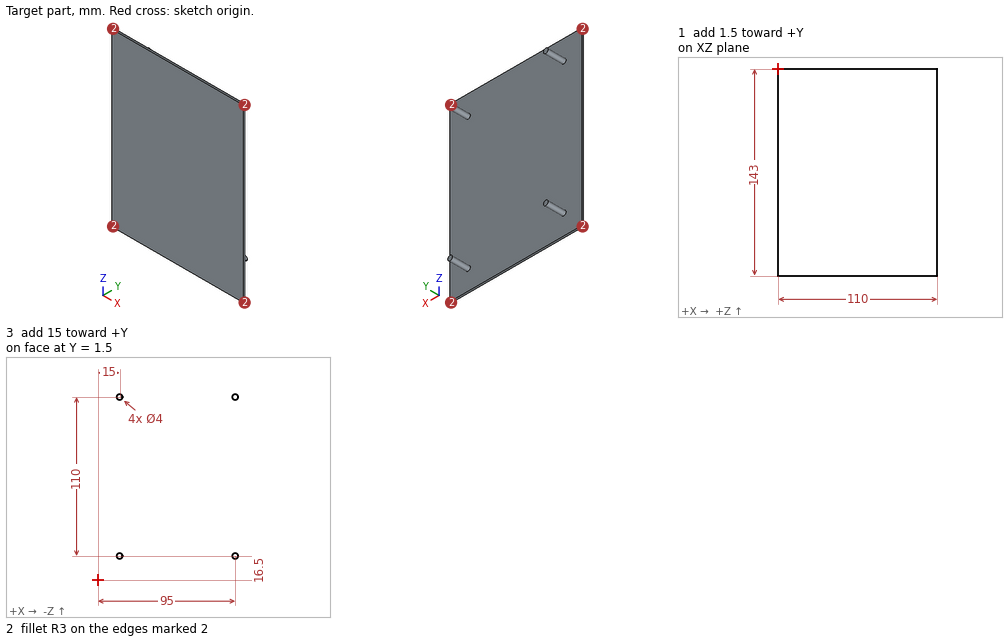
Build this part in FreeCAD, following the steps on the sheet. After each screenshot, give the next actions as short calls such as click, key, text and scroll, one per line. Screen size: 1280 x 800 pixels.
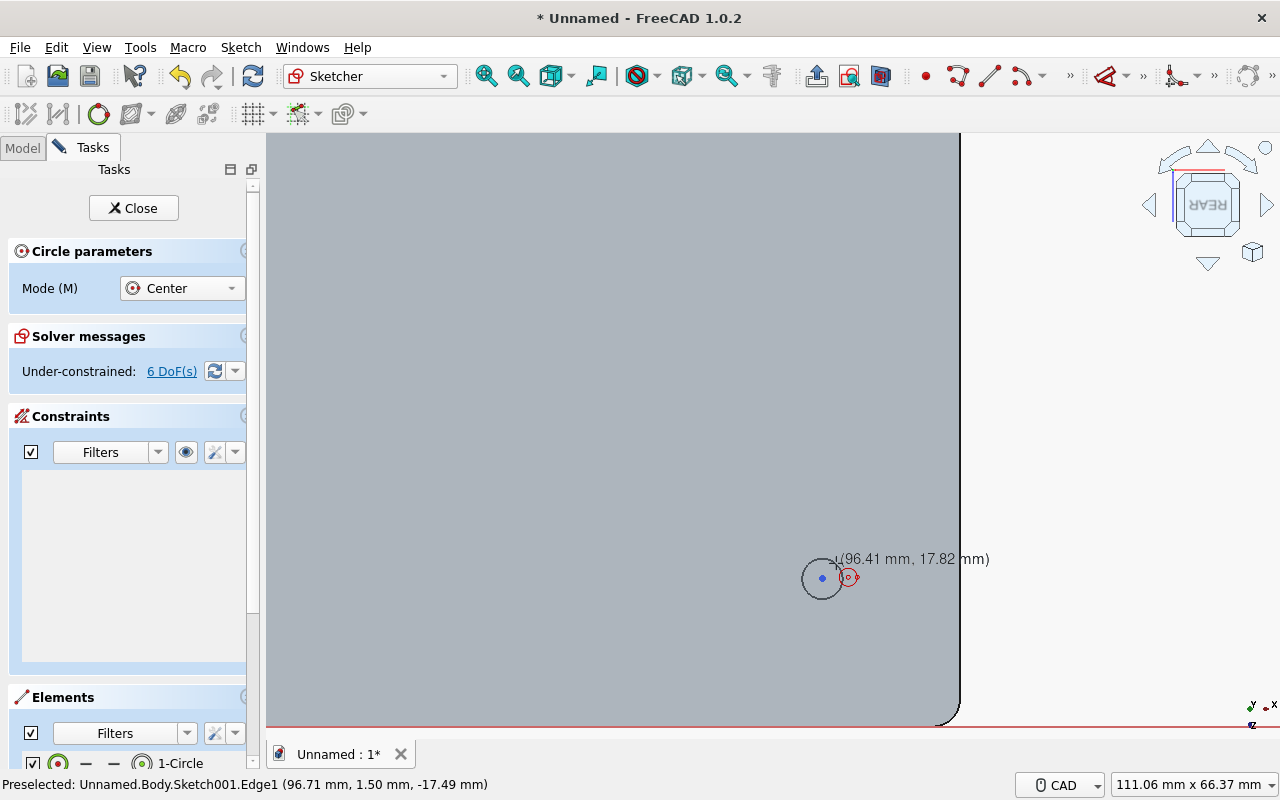
scroll(836, 564, down, 6)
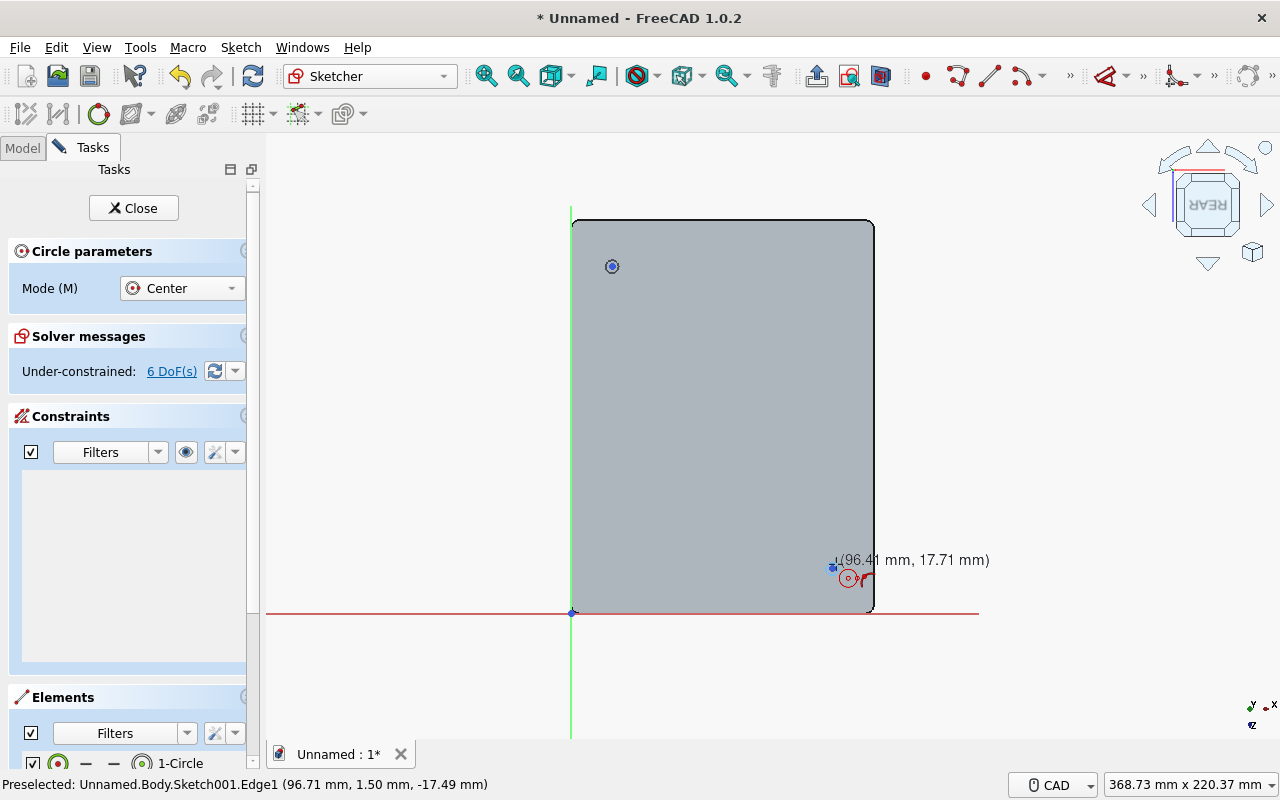
scroll(613, 568, up, 8)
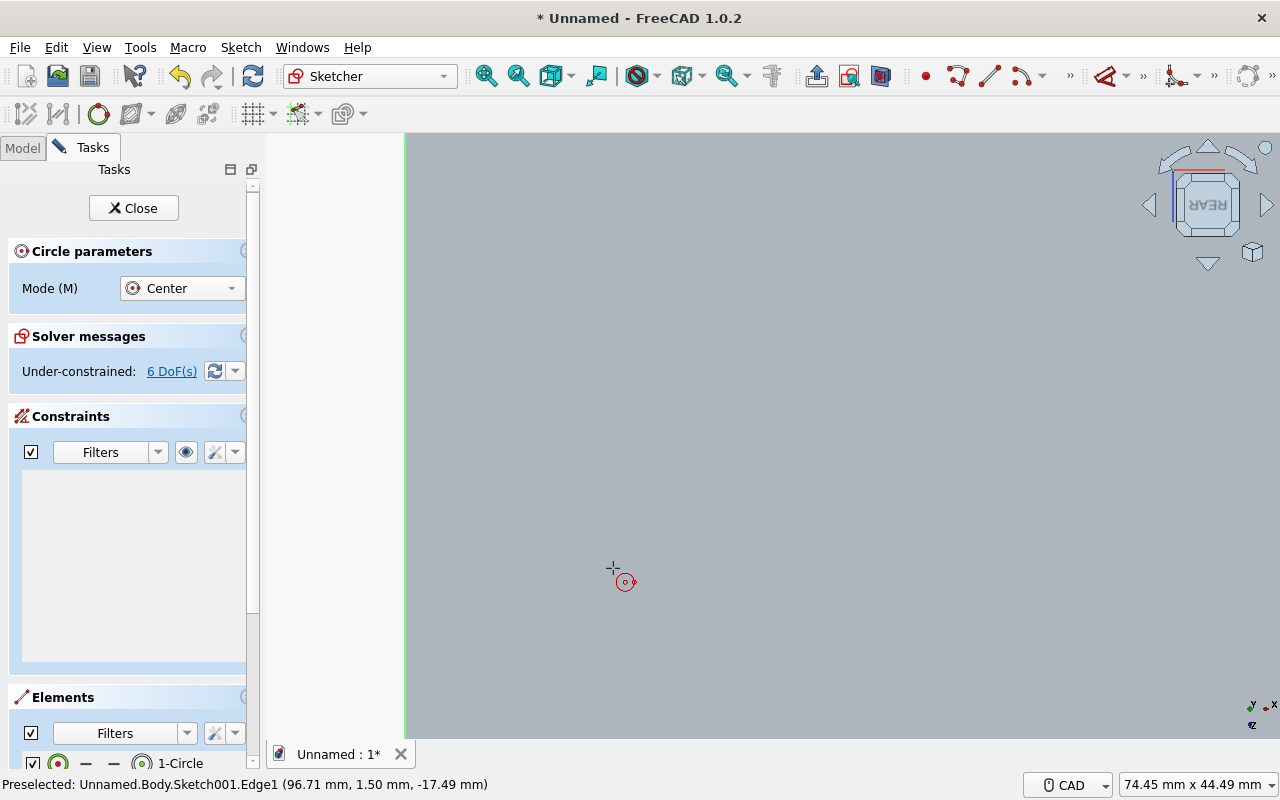
scroll(613, 568, down, 8)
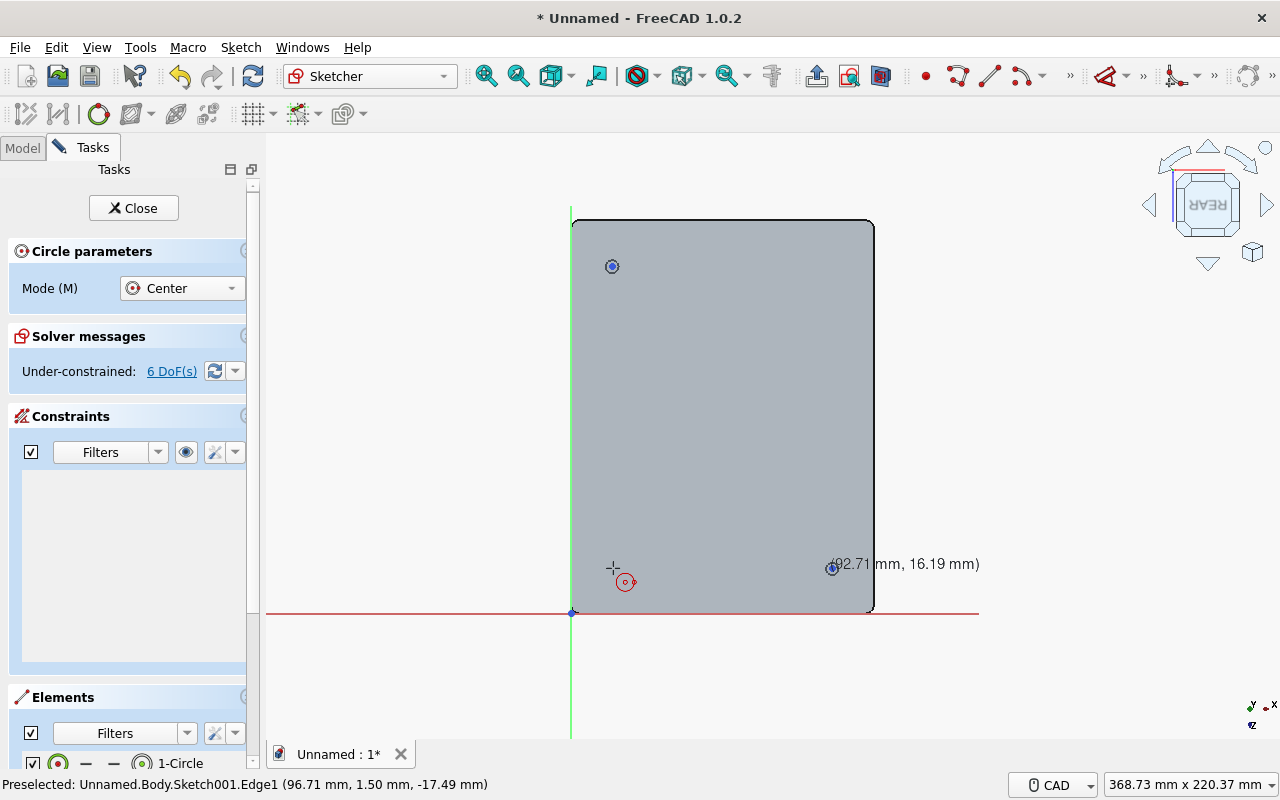
click(613, 568)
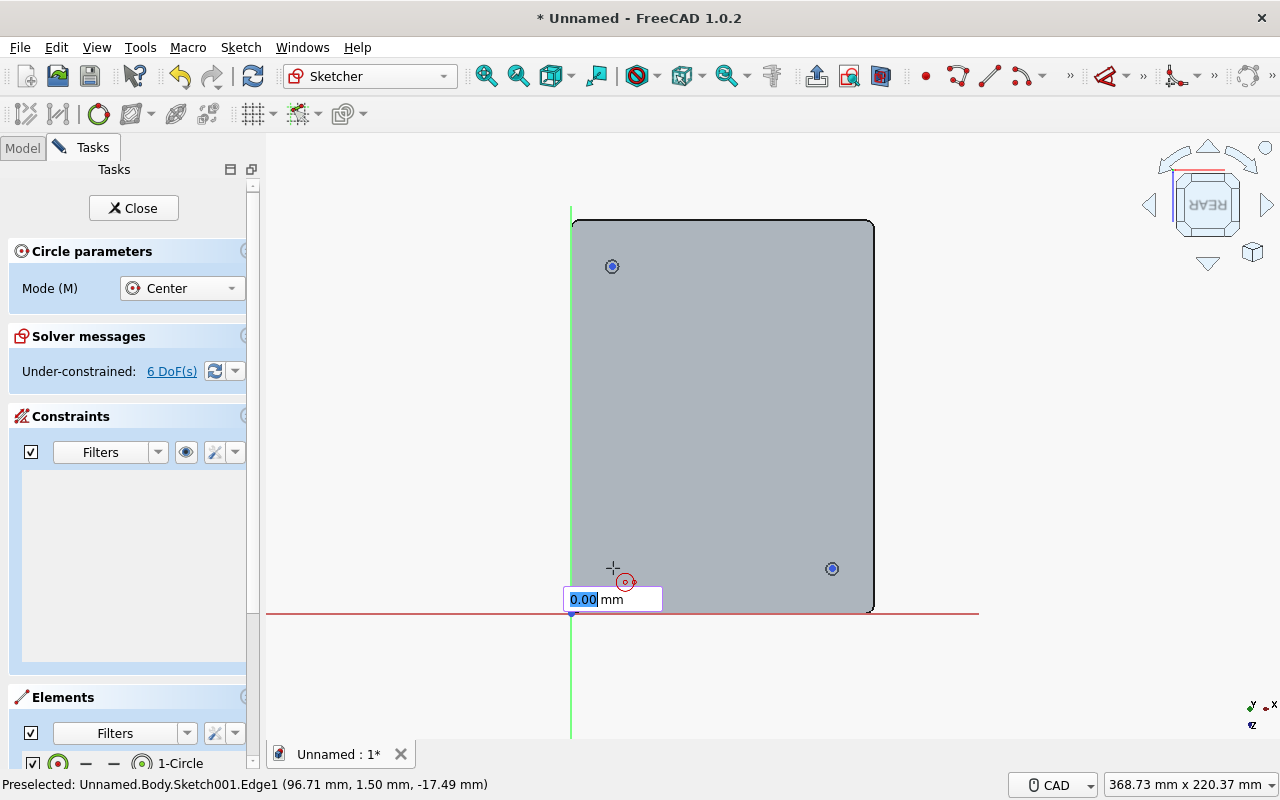
scroll(616, 564, up, 6)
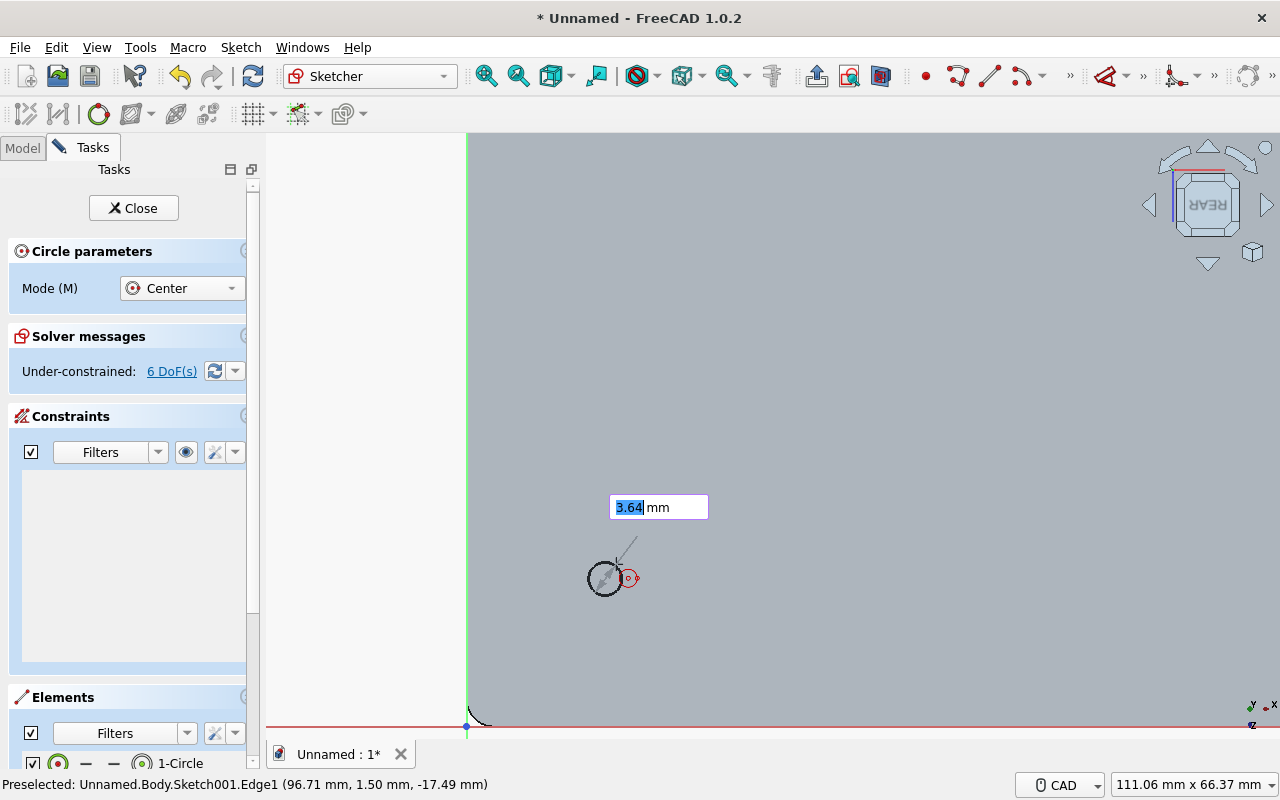
click(617, 563)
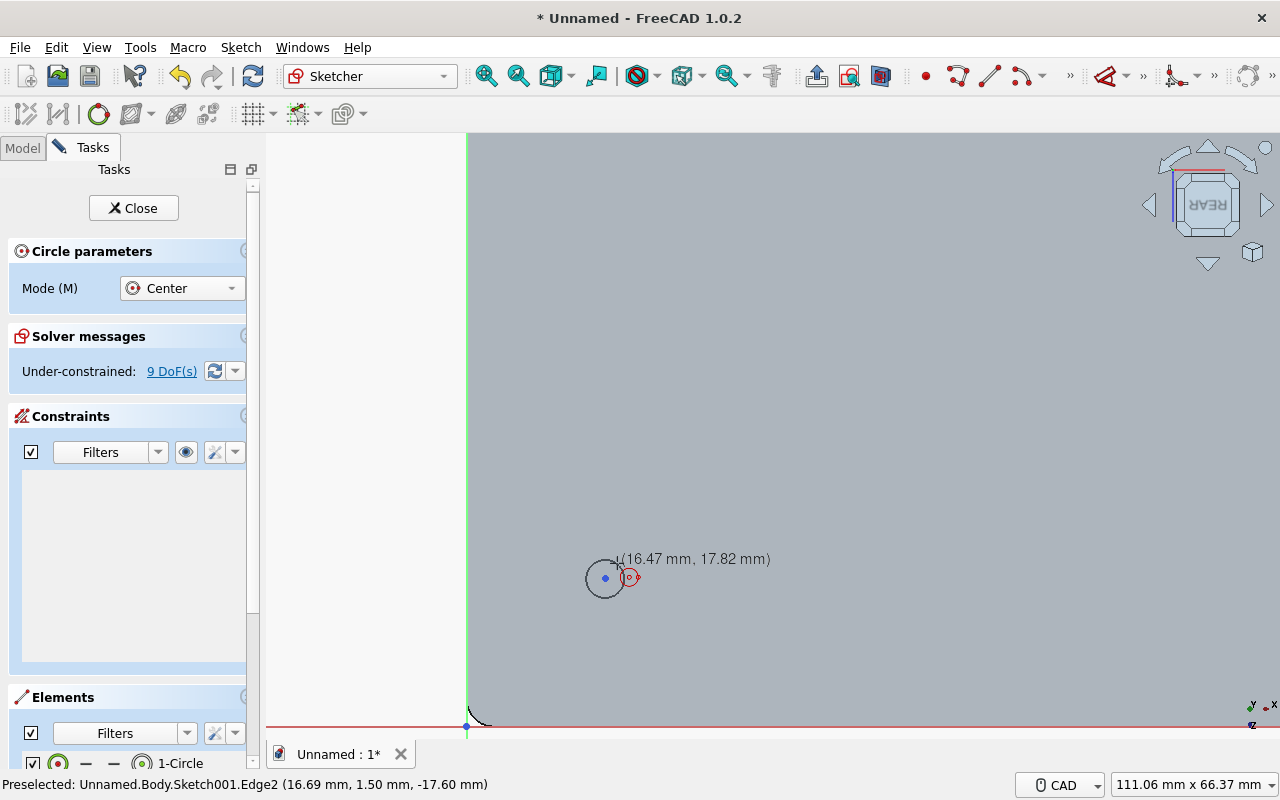
scroll(616, 564, down, 6)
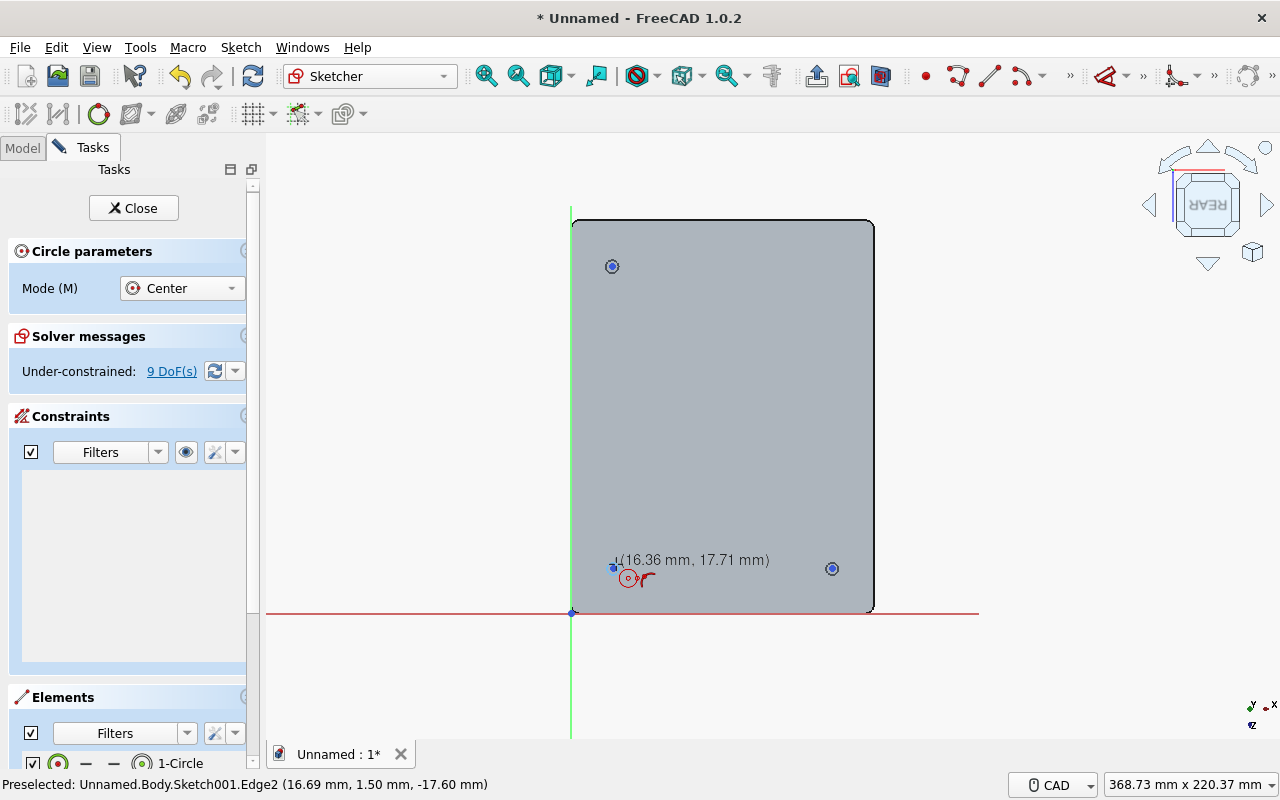
scroll(833, 266, up, 8)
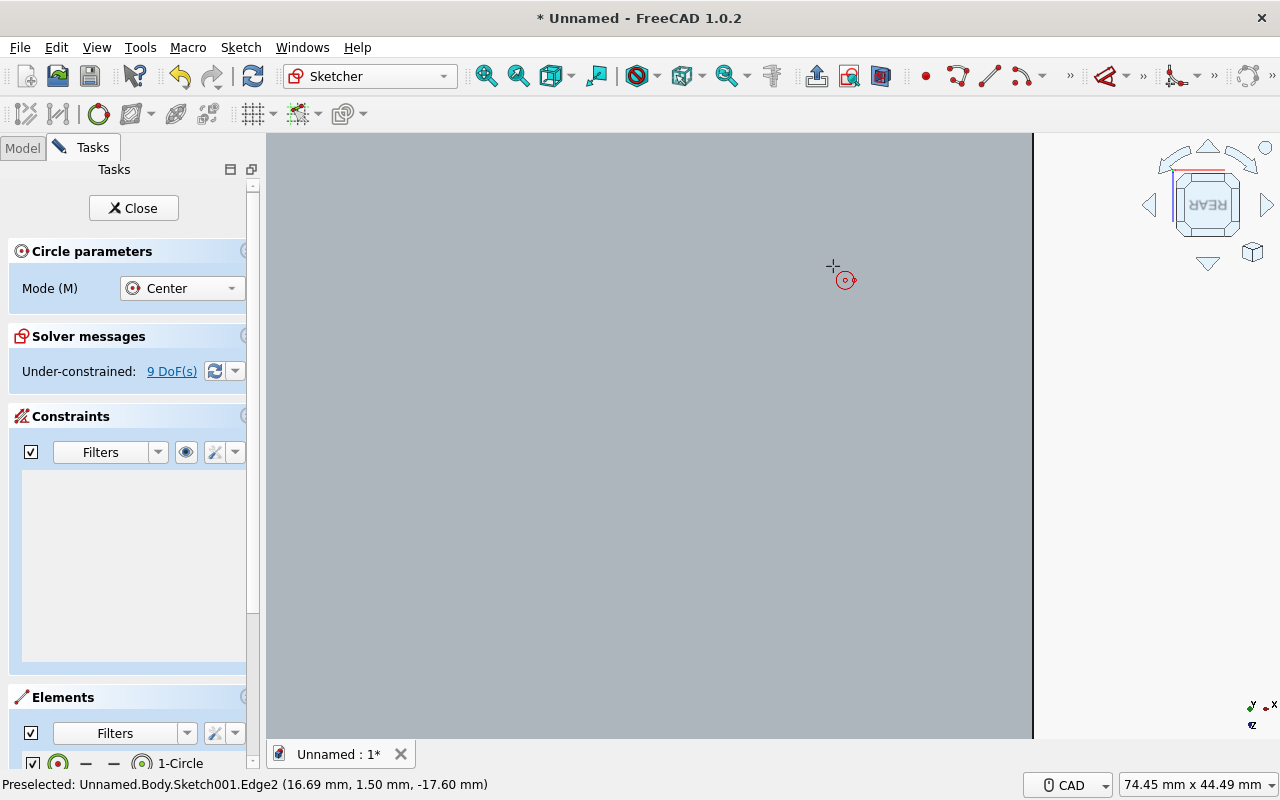
scroll(833, 265, down, 8)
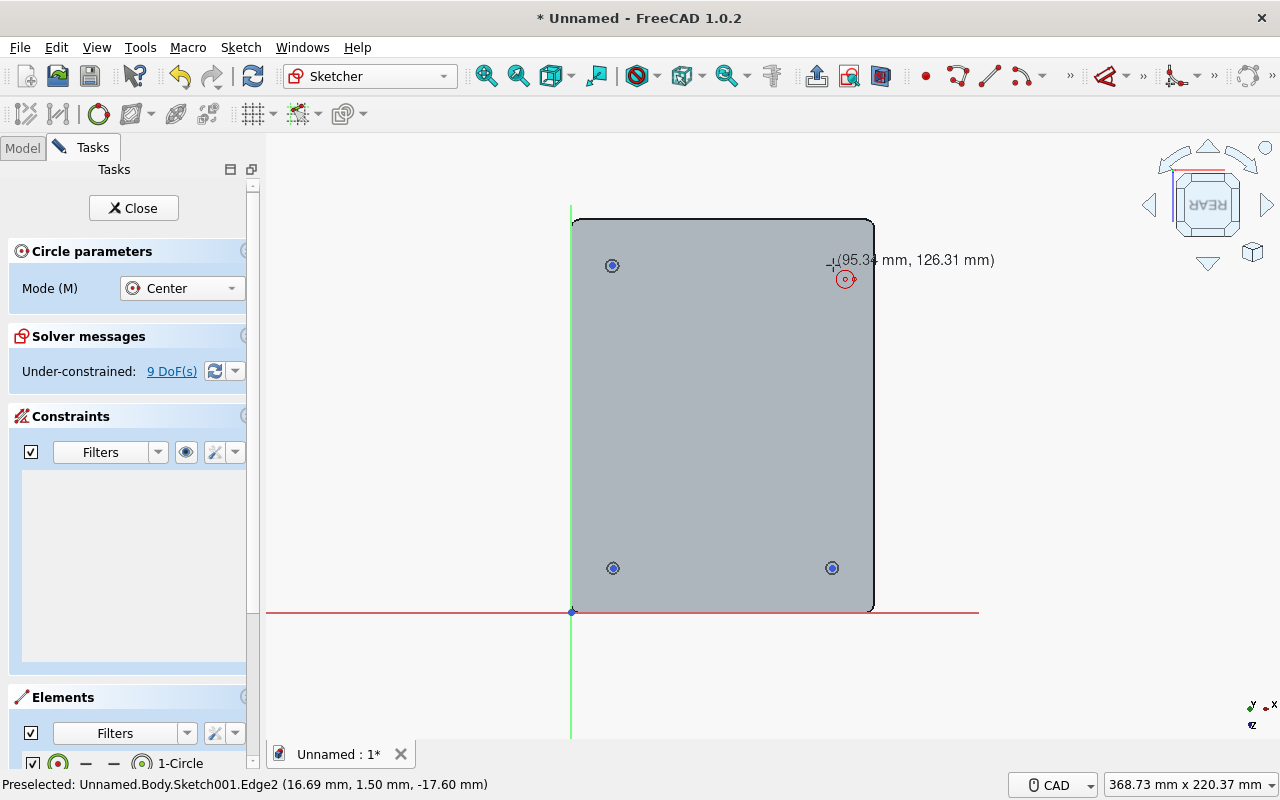
click(833, 265)